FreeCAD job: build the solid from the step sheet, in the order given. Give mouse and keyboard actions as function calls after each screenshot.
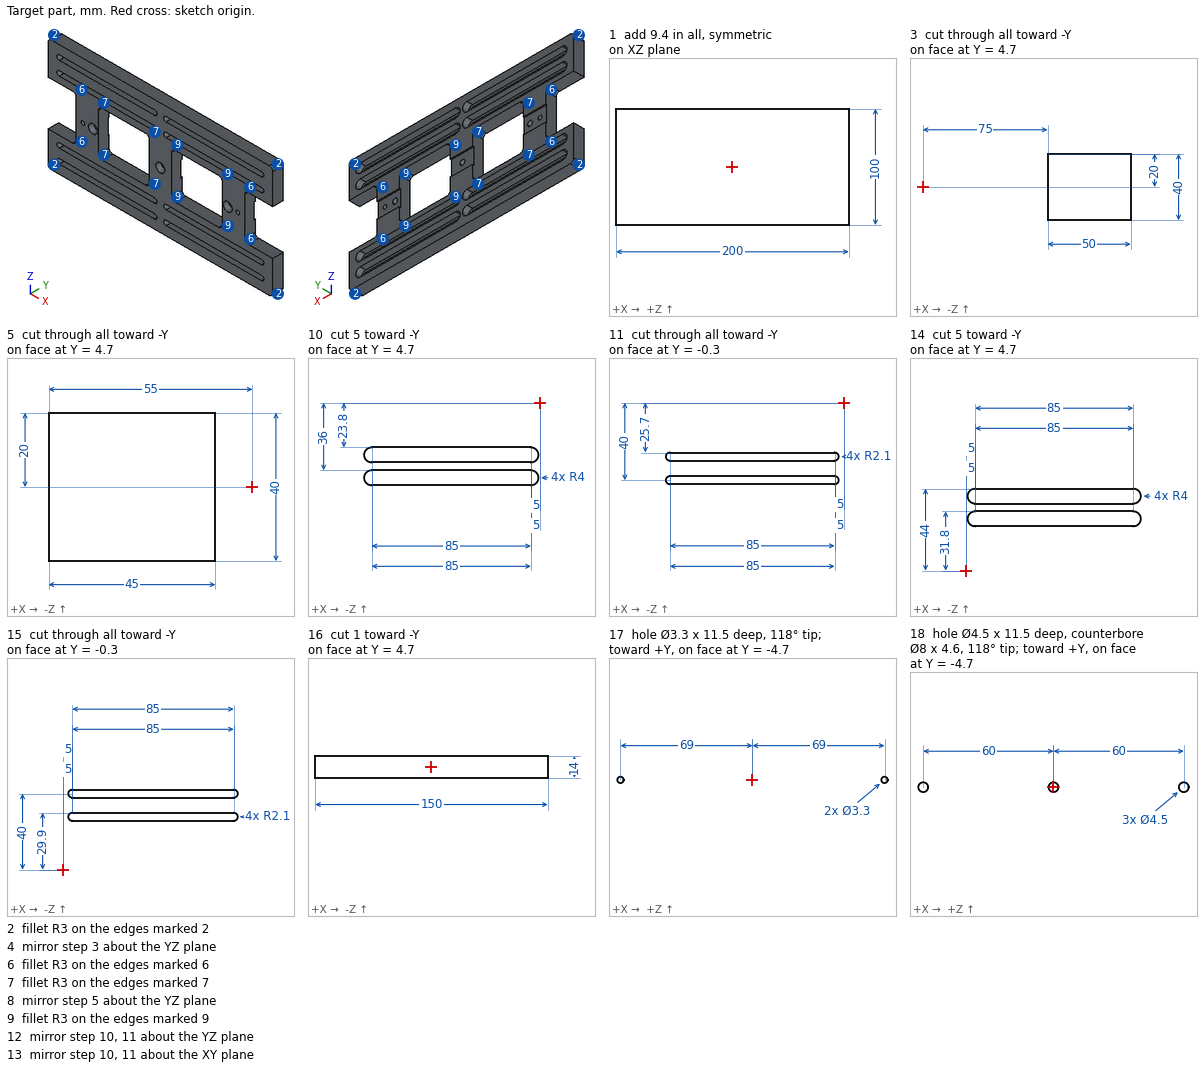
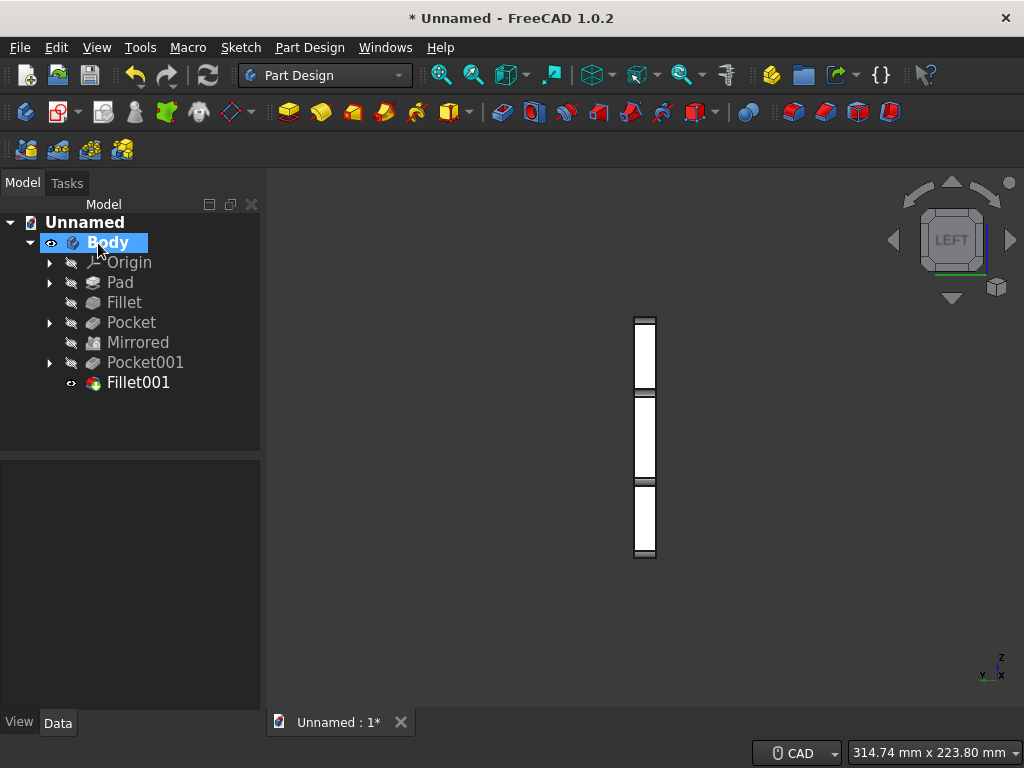
key(0)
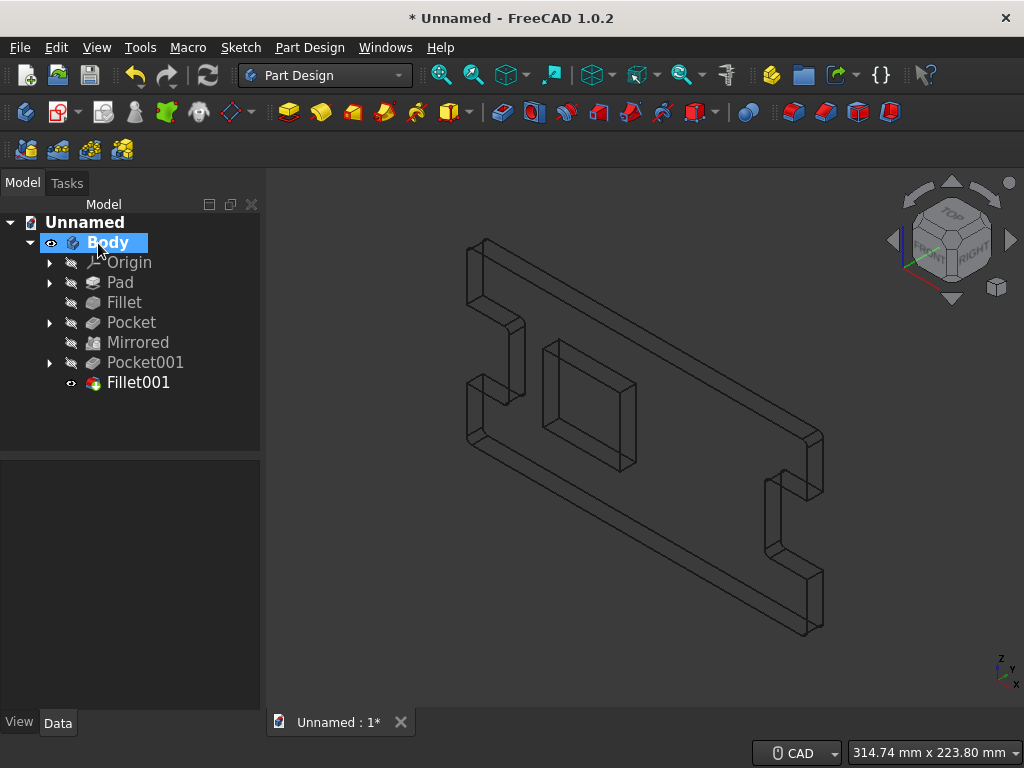
click(551, 343)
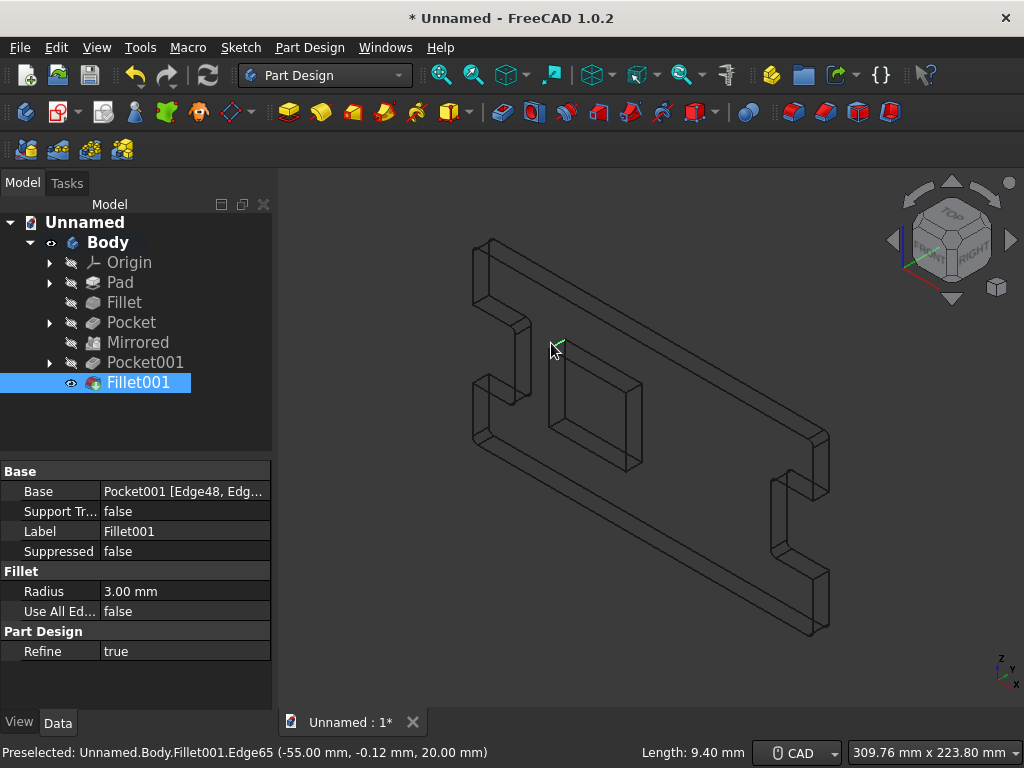
click(557, 422, ctrl)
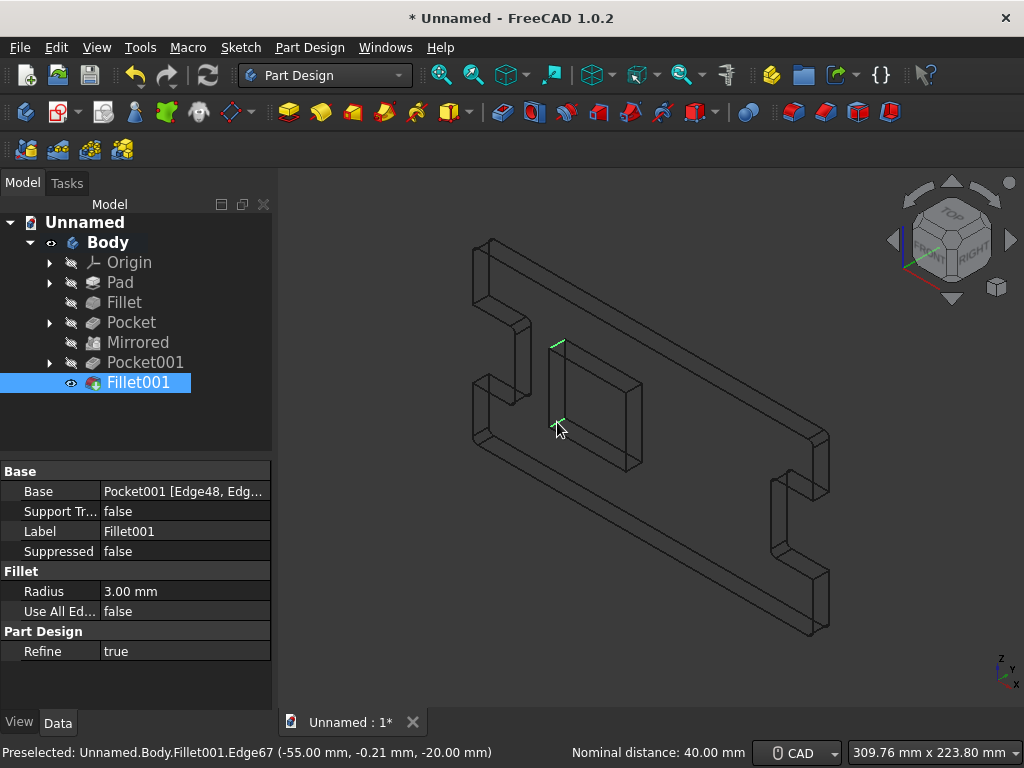
click(634, 466, ctrl)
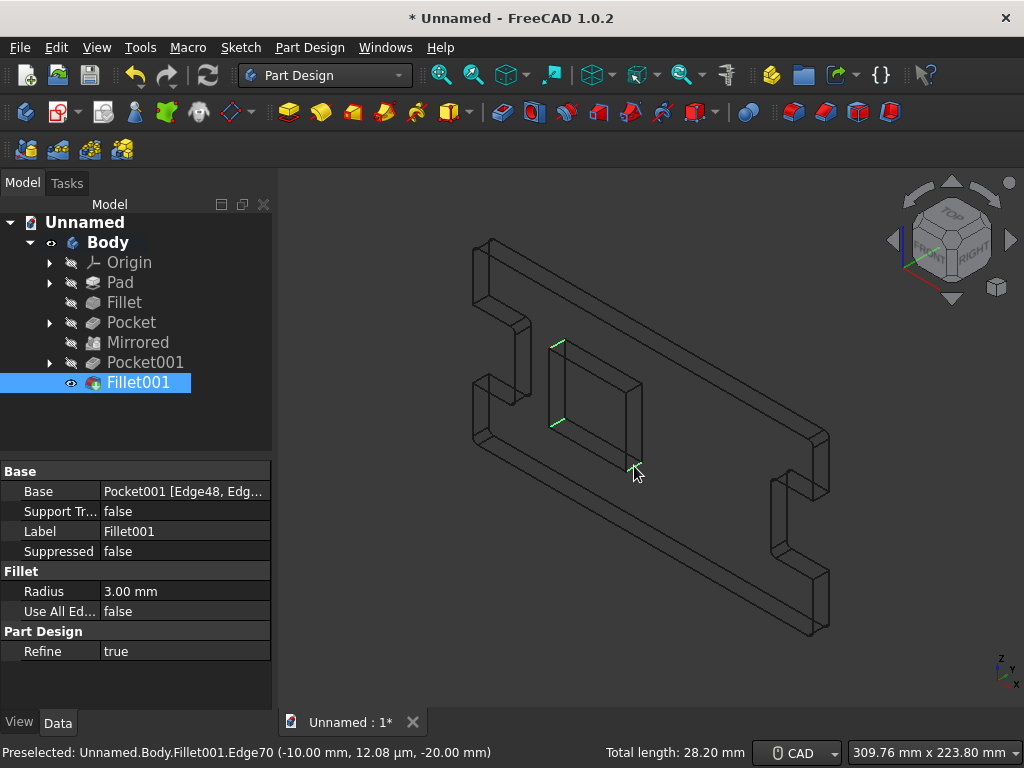
click(634, 387, ctrl)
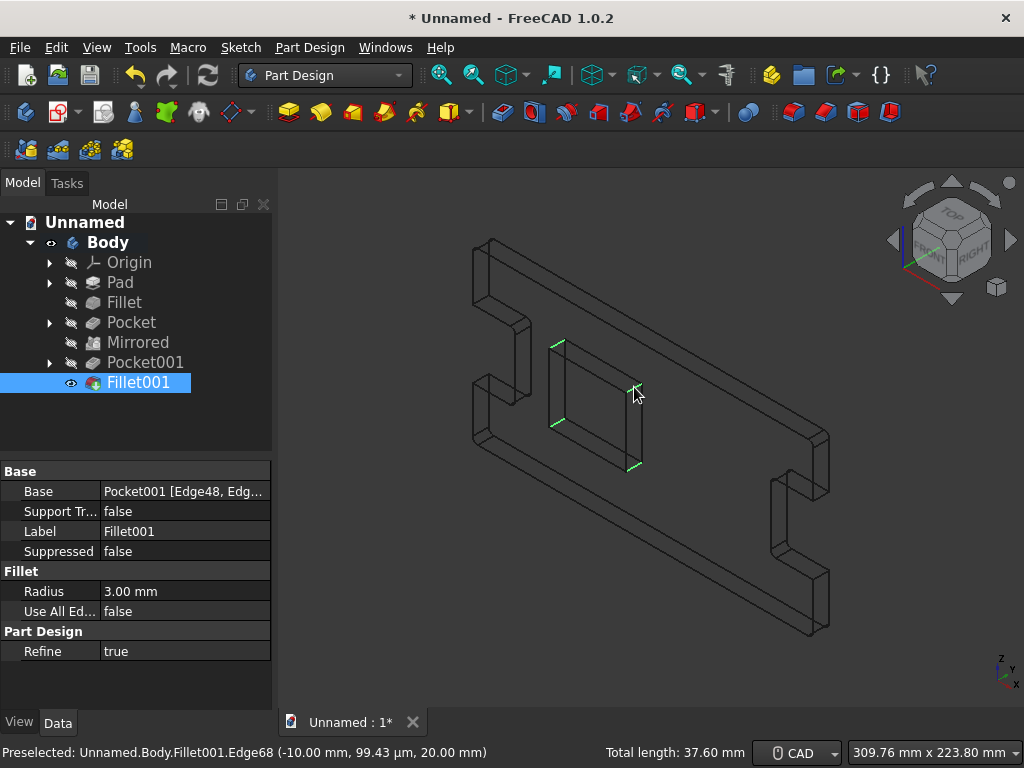
key(v)
key(1)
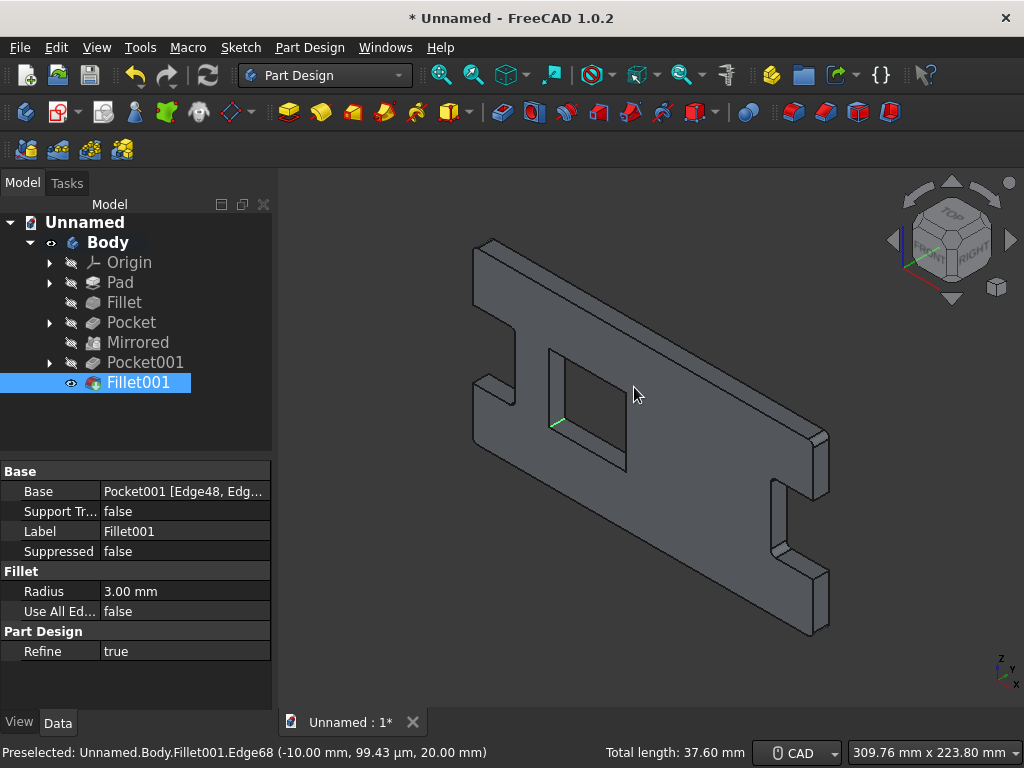
click(794, 112)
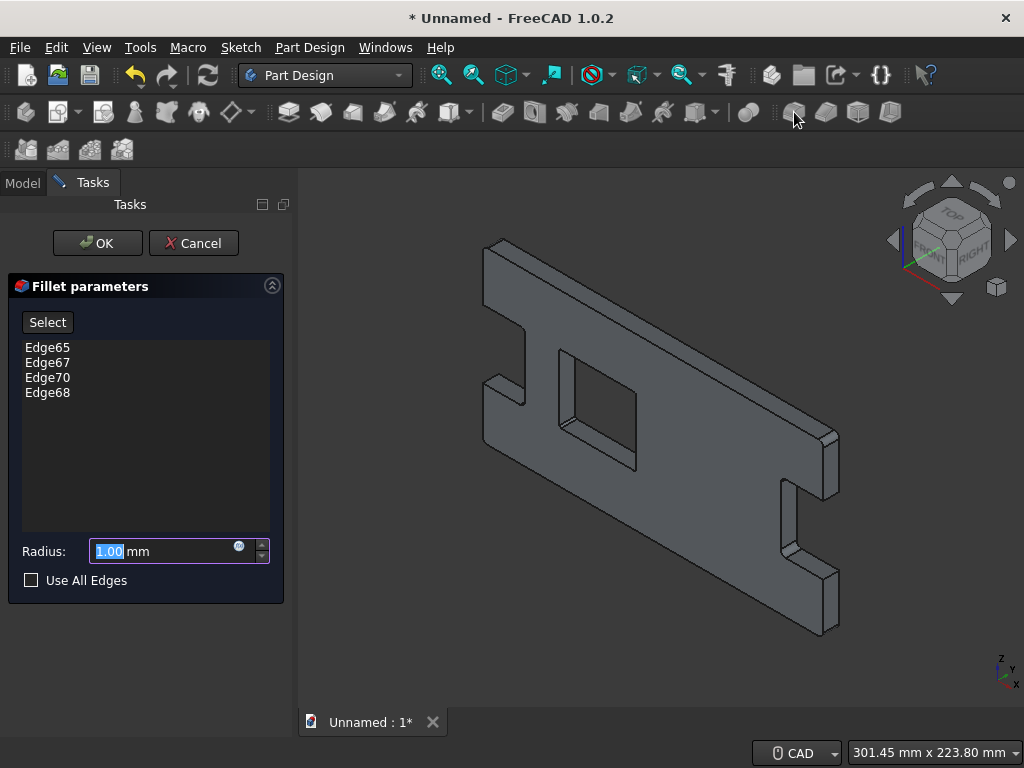
text(3)
key(Tab)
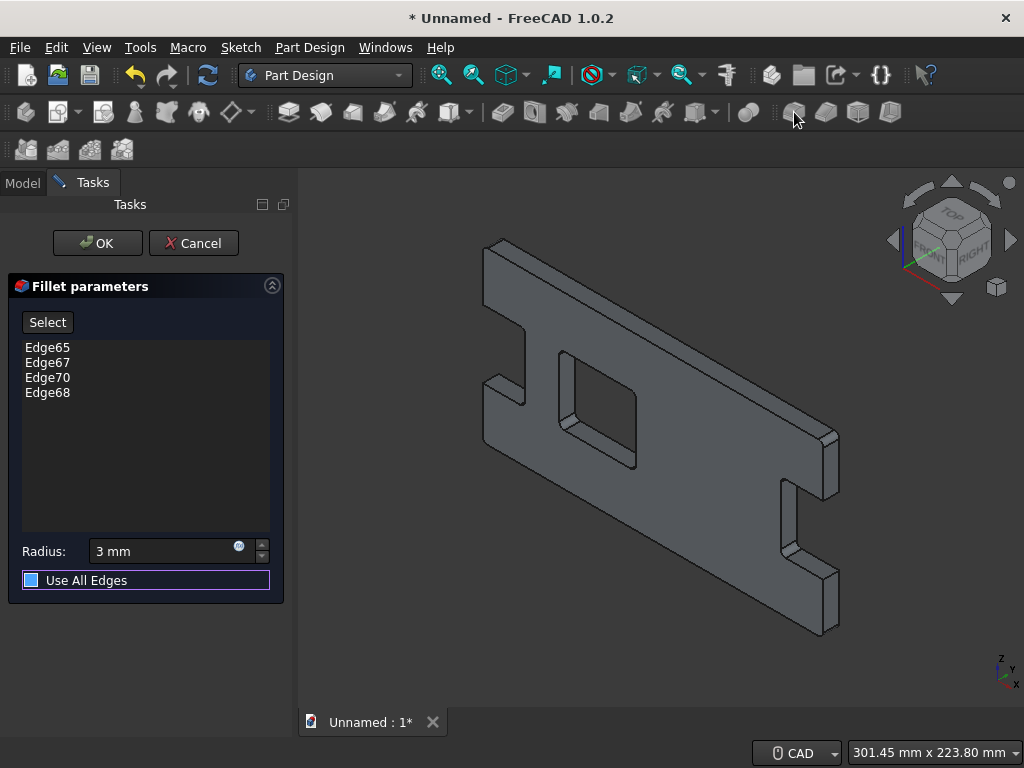
click(98, 243)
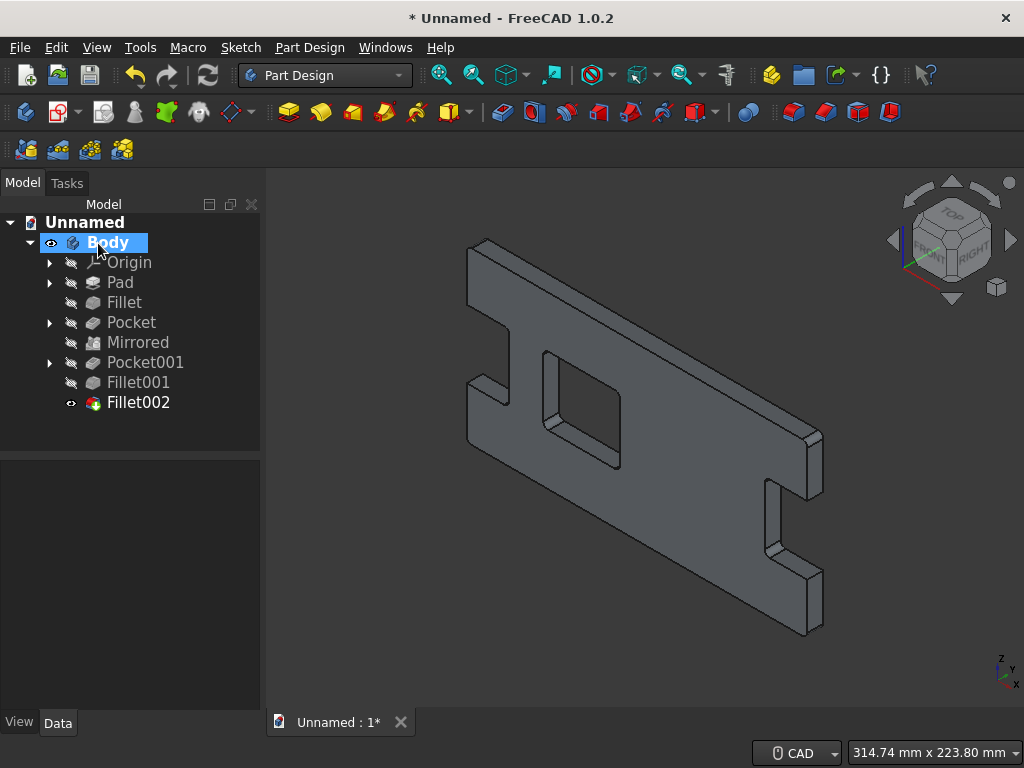
click(116, 363)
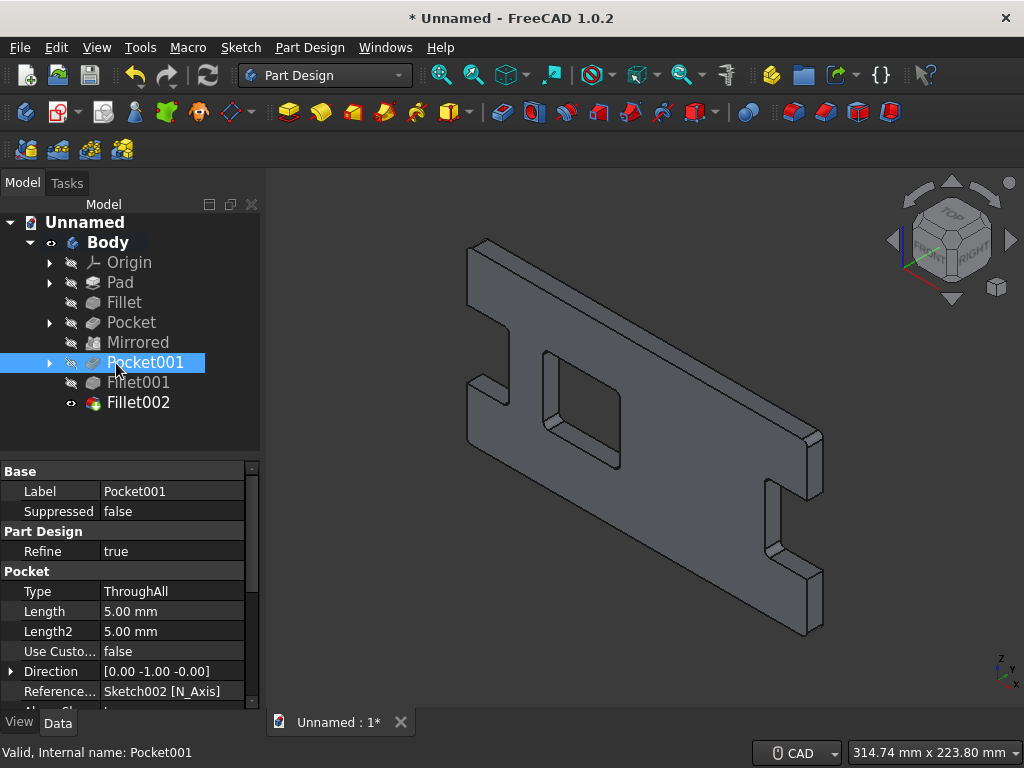
click(26, 150)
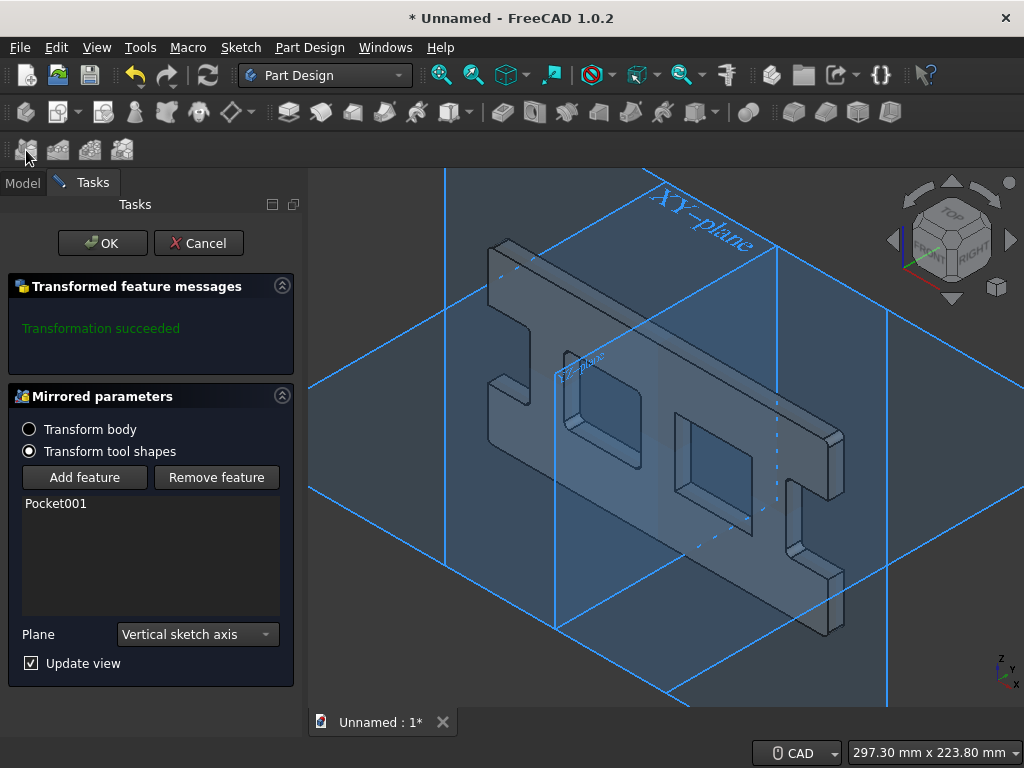
click(198, 634)